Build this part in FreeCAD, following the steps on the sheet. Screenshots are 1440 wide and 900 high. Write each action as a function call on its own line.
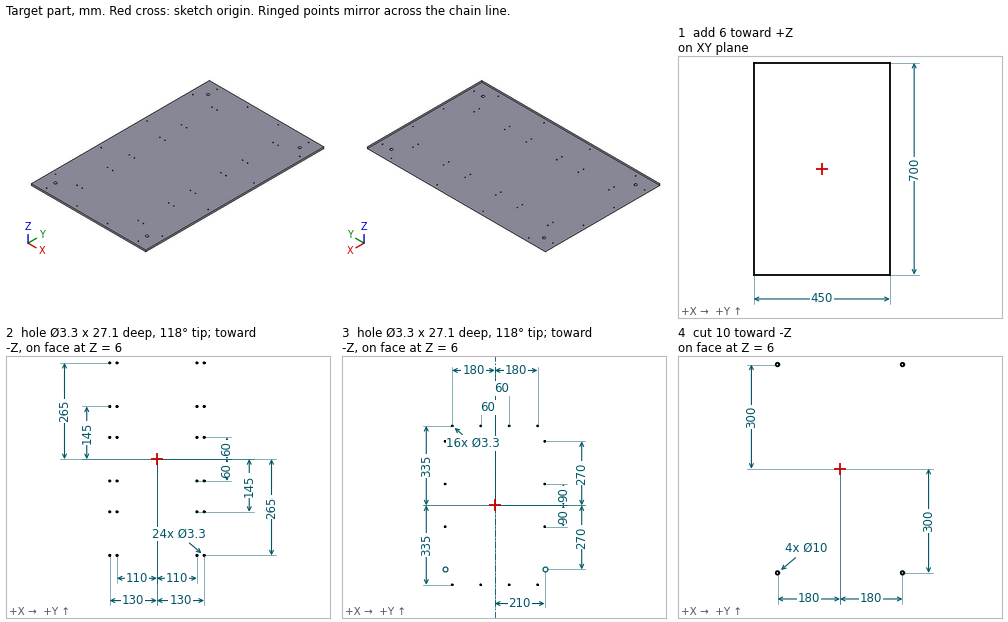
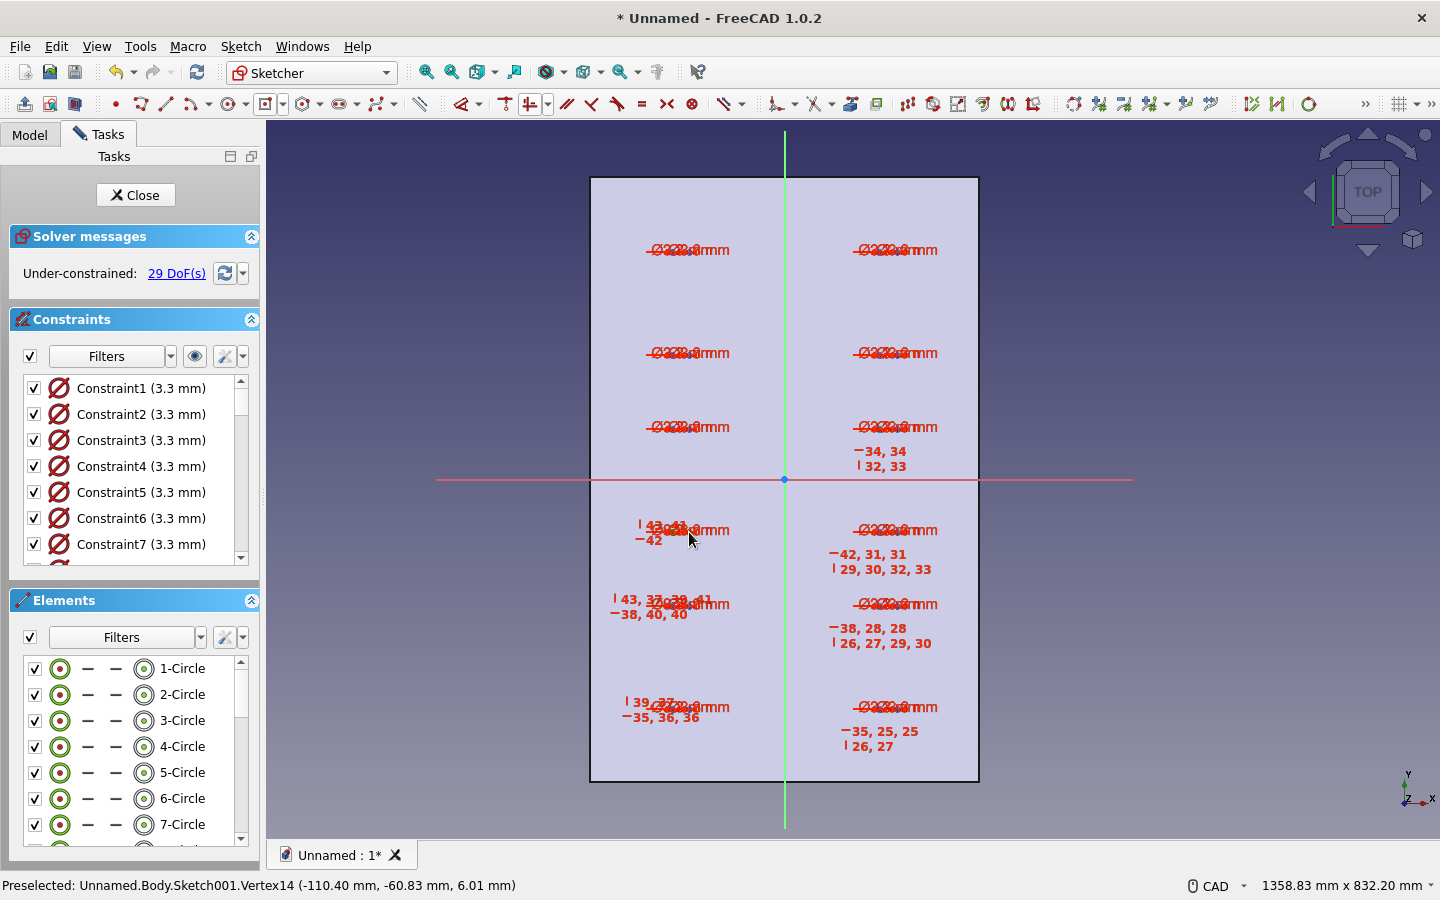
click(548, 104)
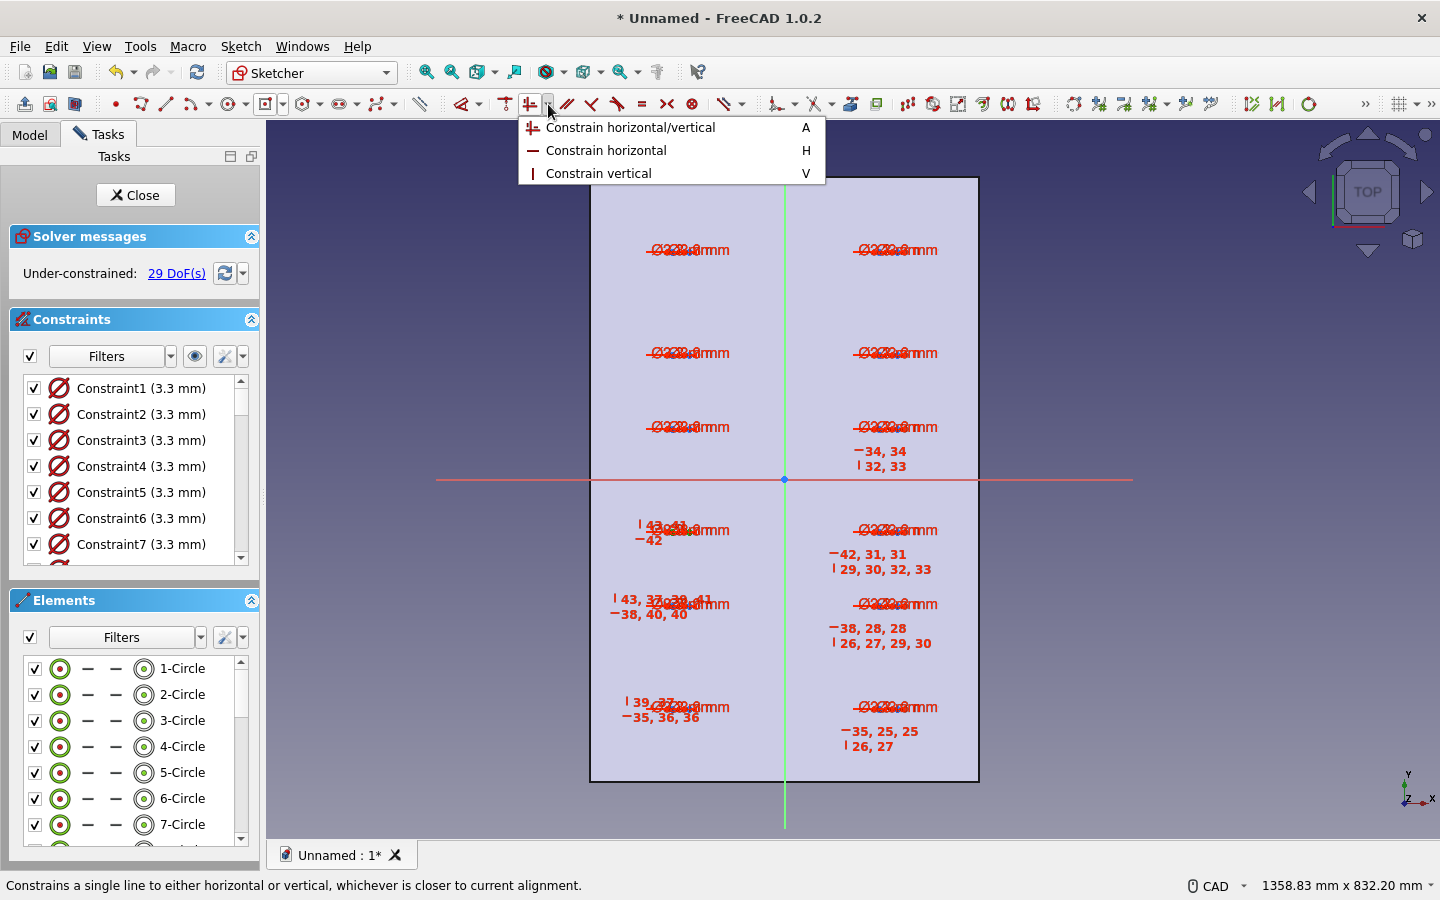
click(672, 150)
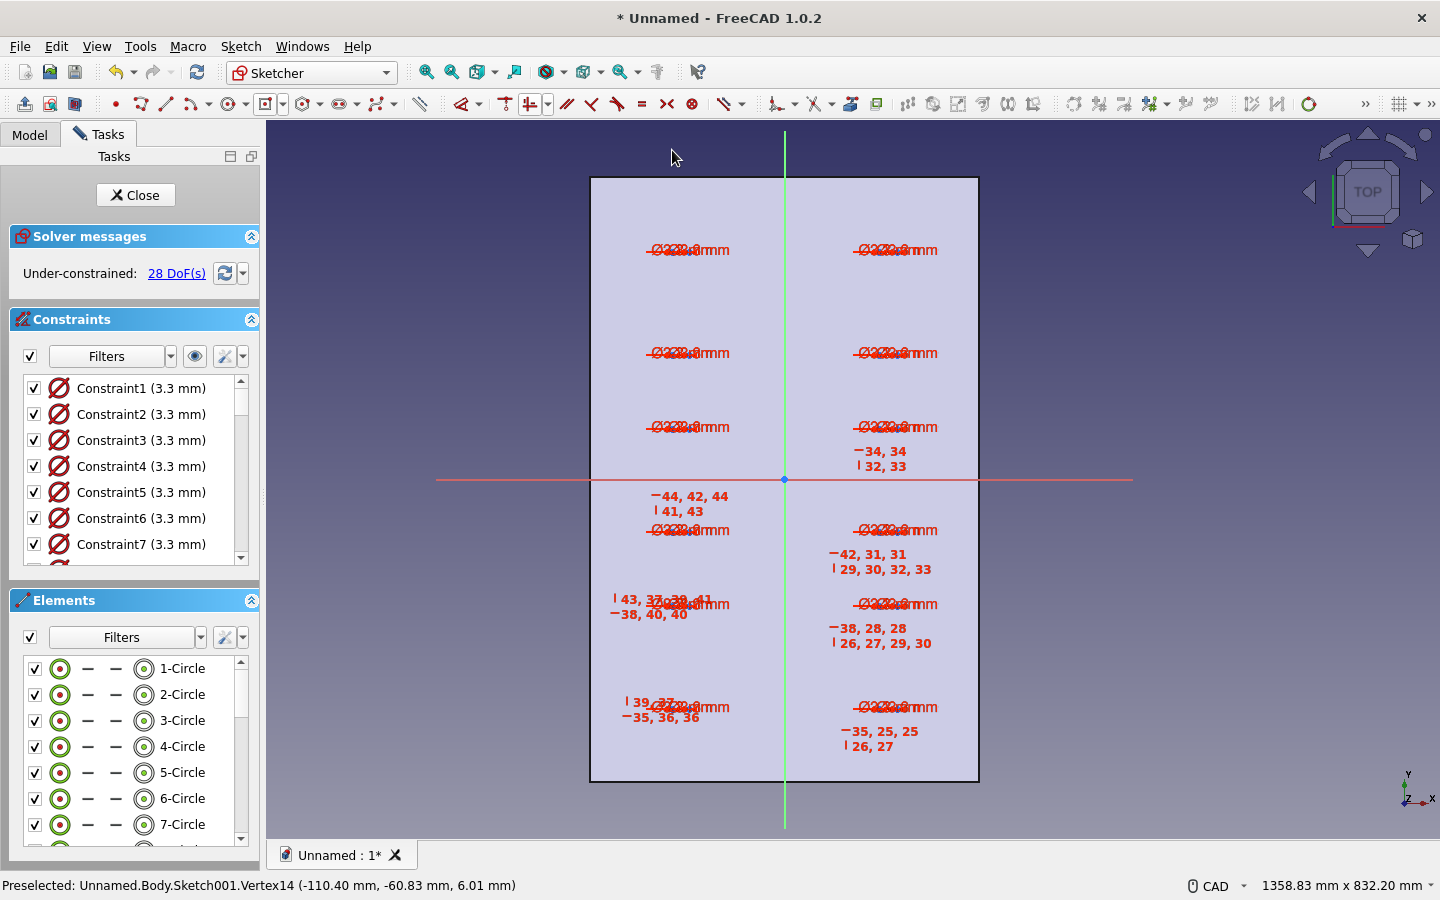
click(672, 532)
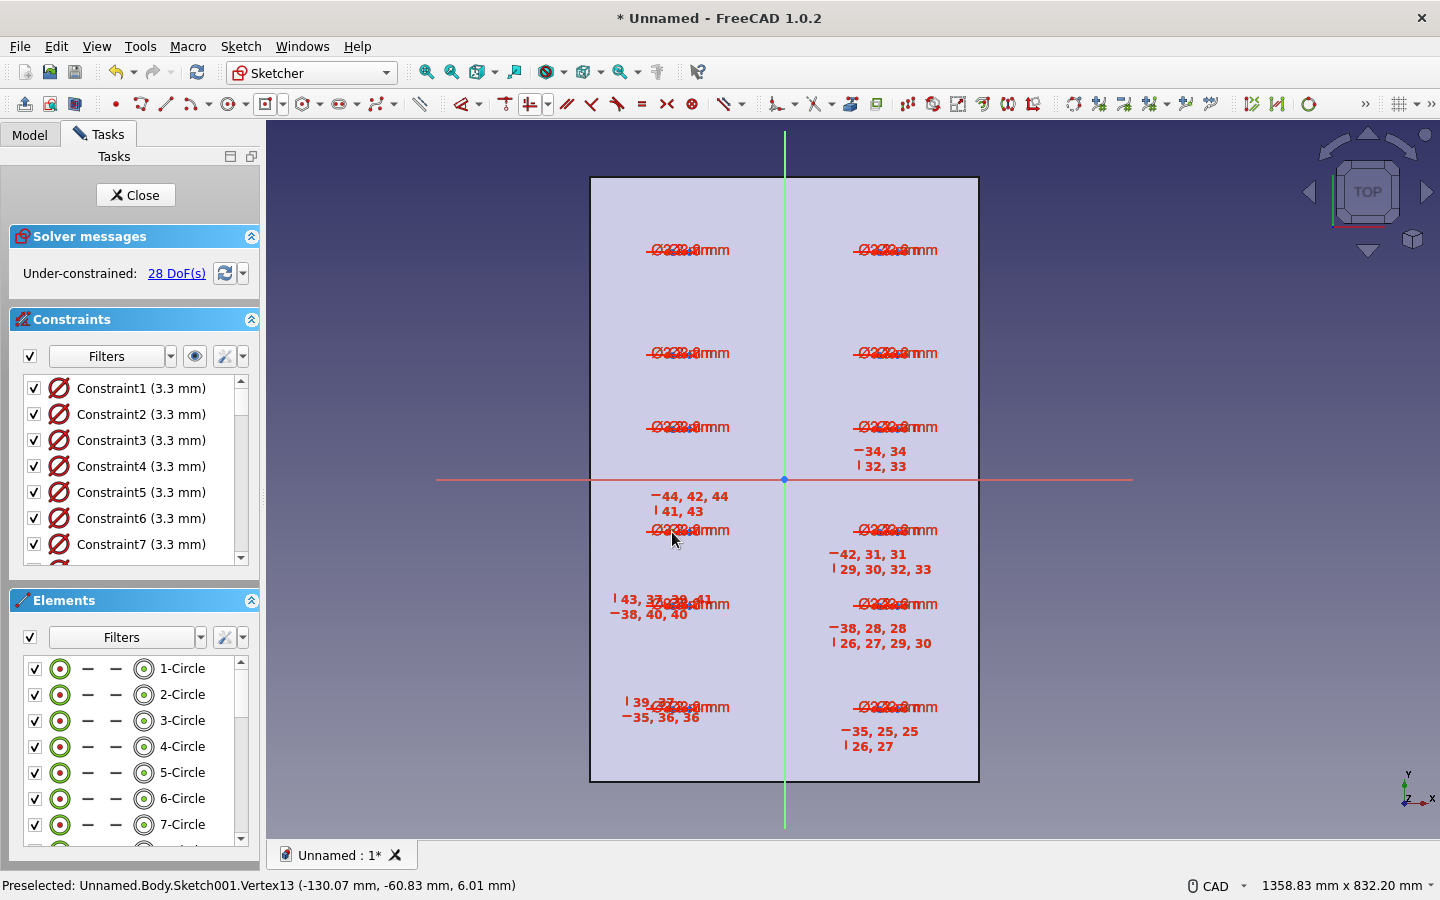
click(672, 429)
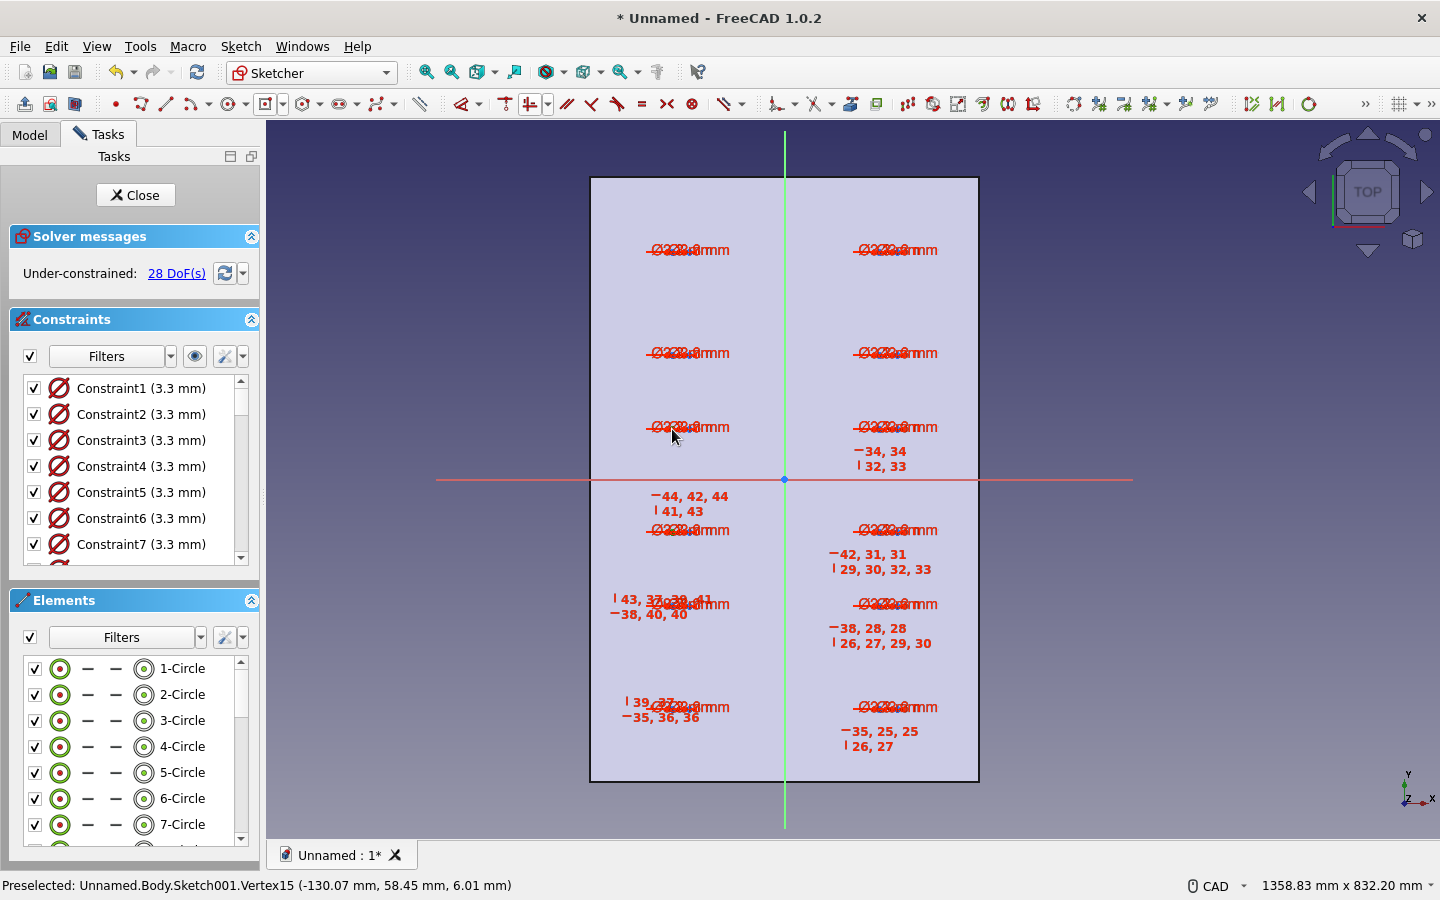
click(548, 104)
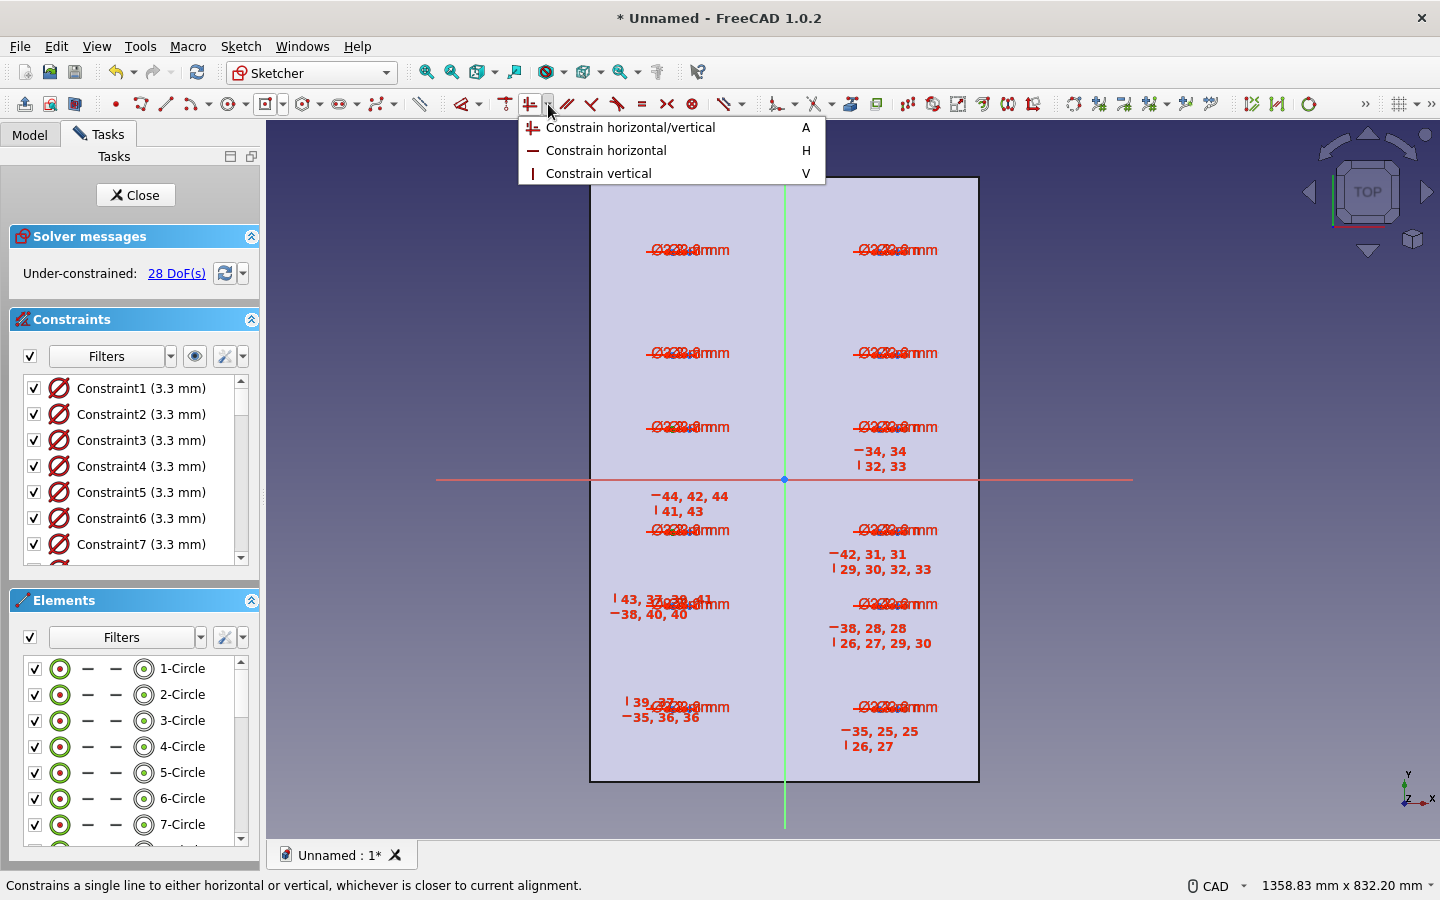
click(672, 174)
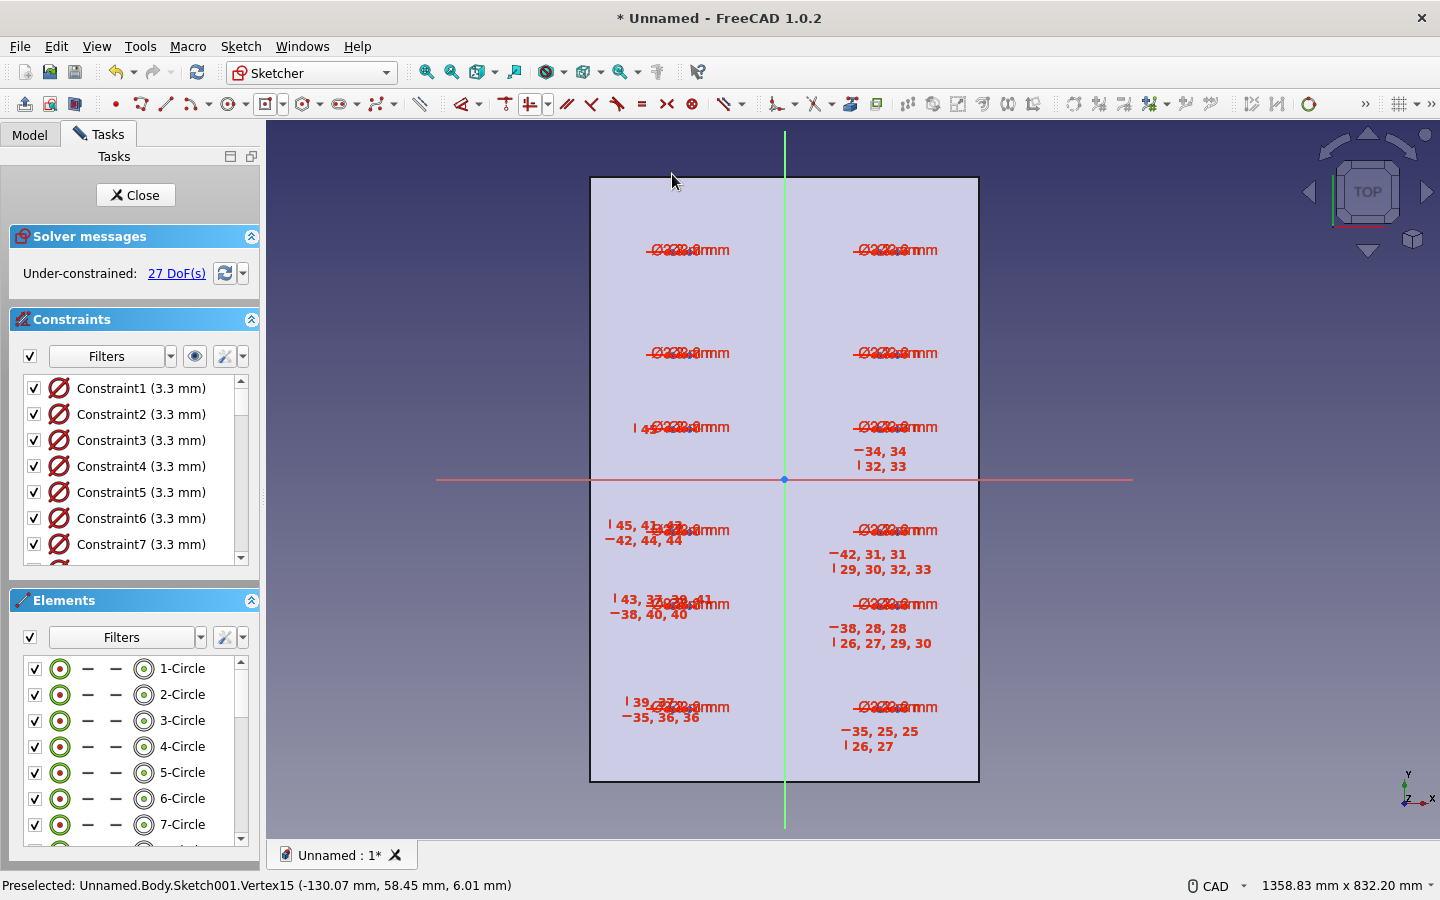
click(879, 429)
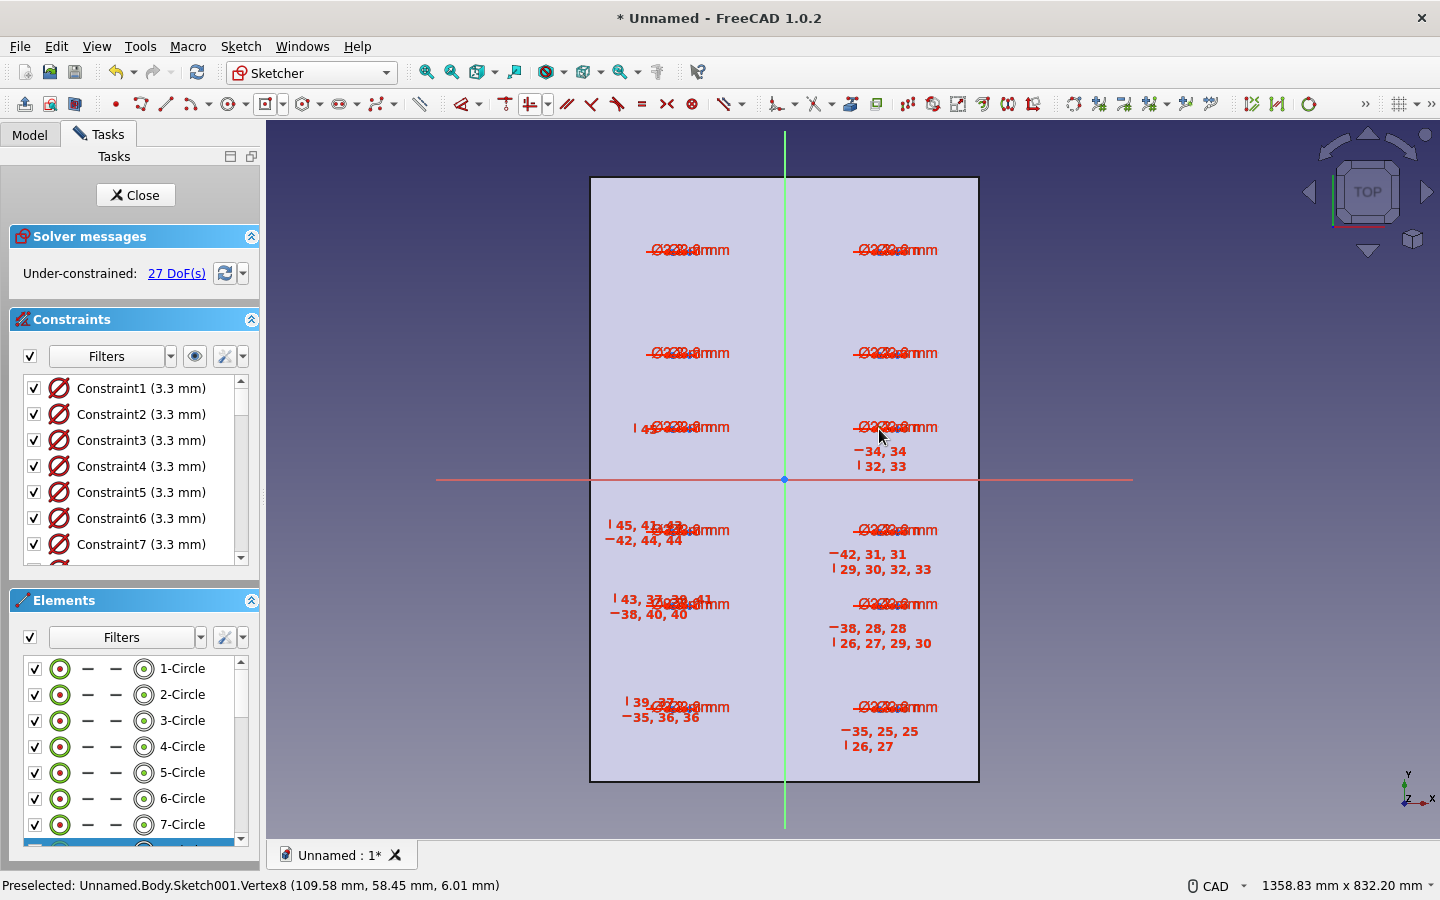
click(672, 429)